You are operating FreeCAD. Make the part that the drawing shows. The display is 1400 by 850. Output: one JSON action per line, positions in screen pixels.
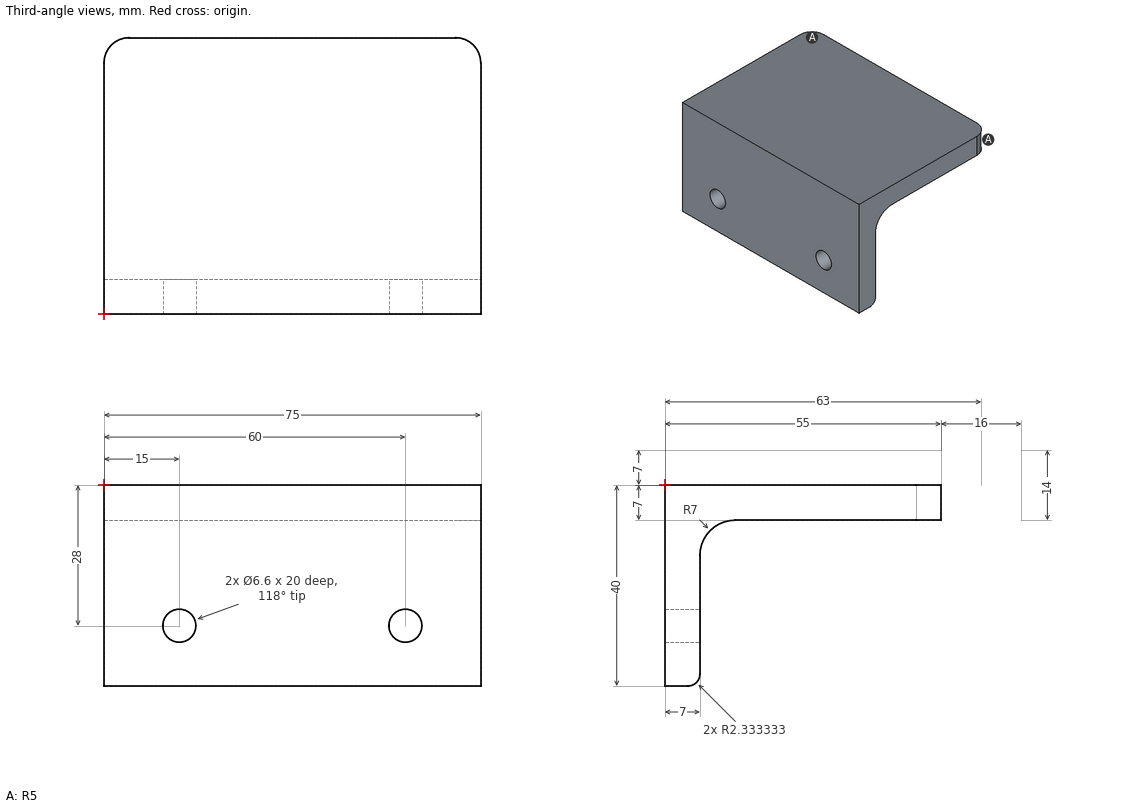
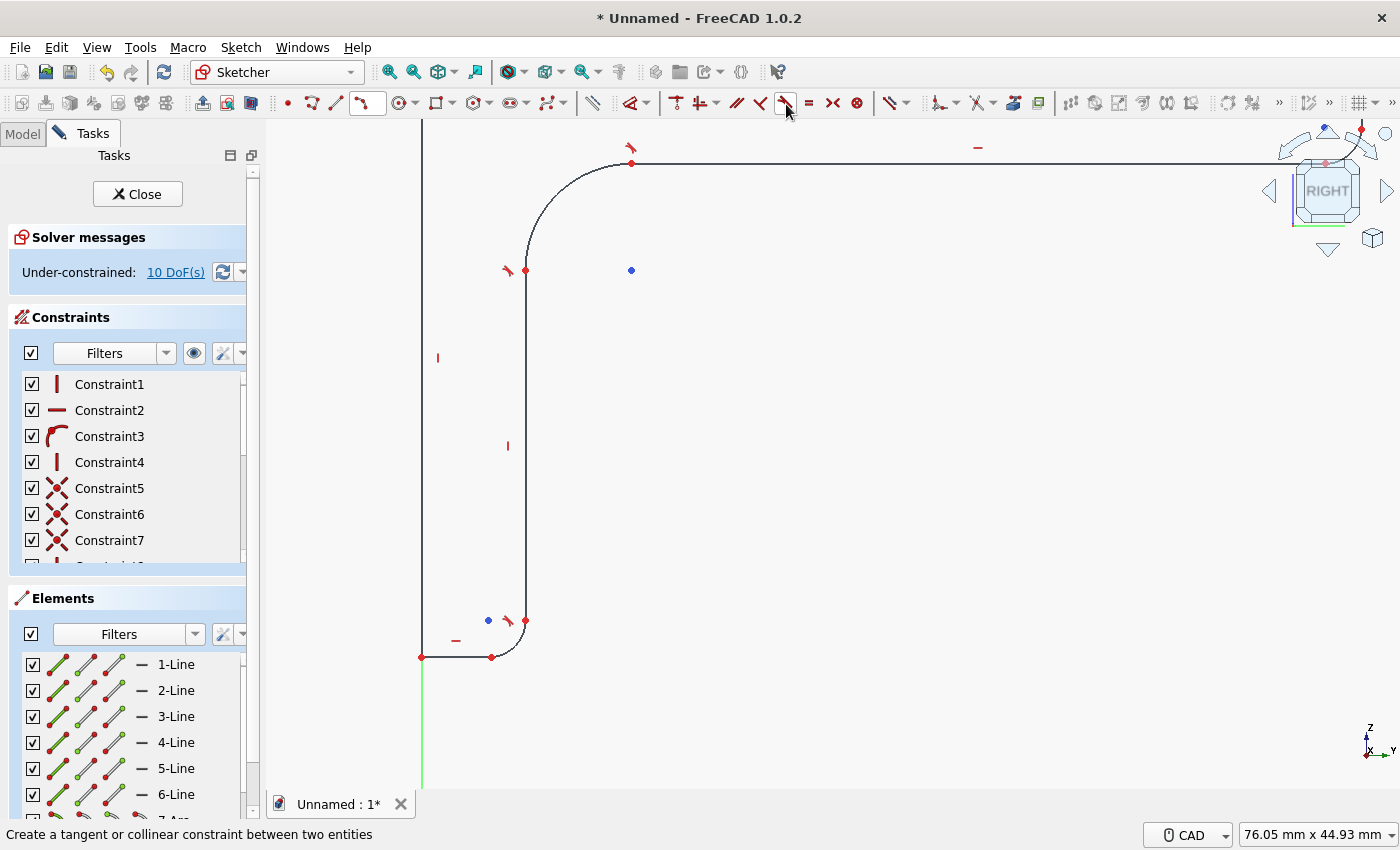
{"action": "left_click", "coordinate": [840, 164]}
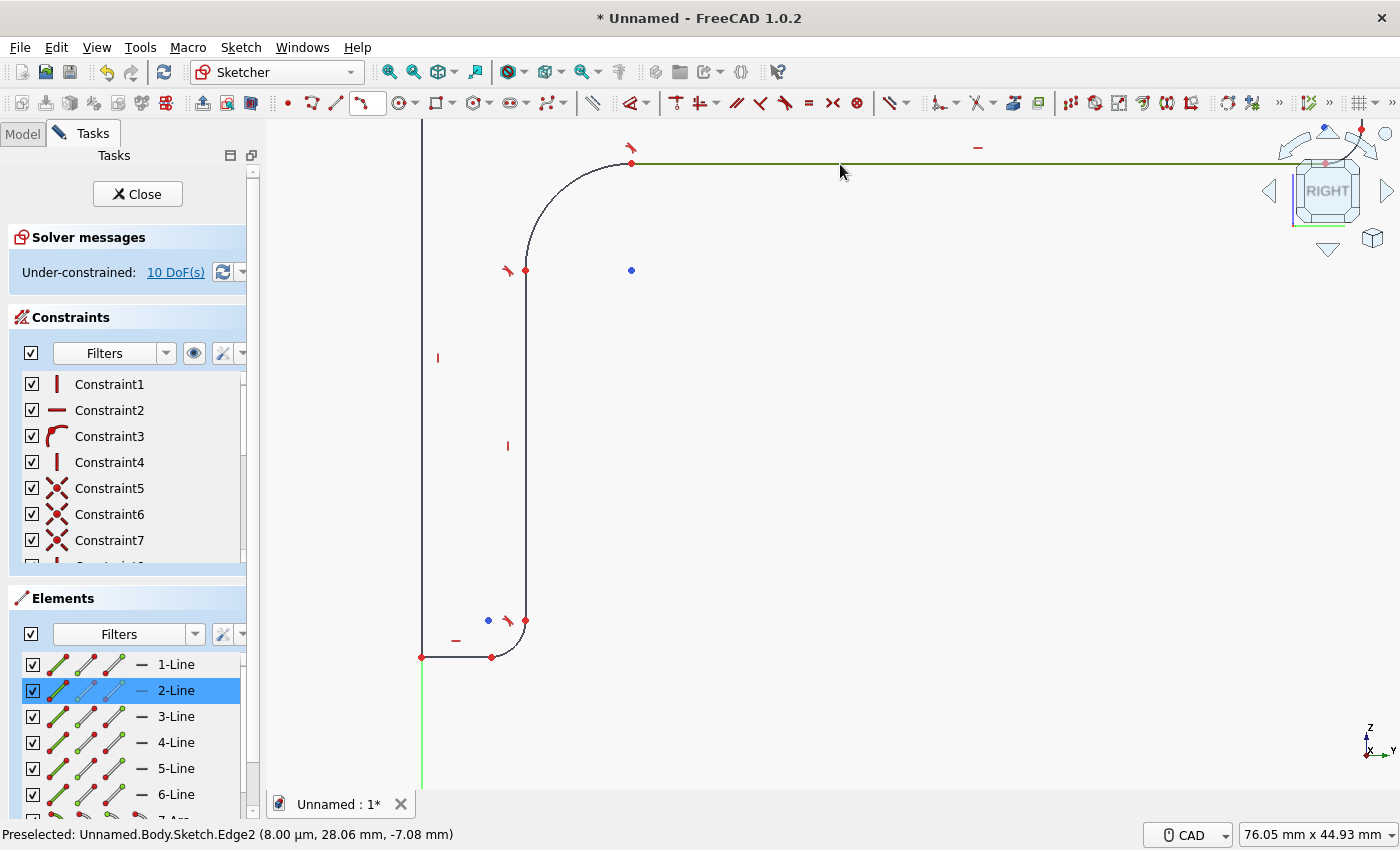
{"action": "scroll", "coordinate": [507, 652], "scroll_direction": "down", "scroll_amount": 2}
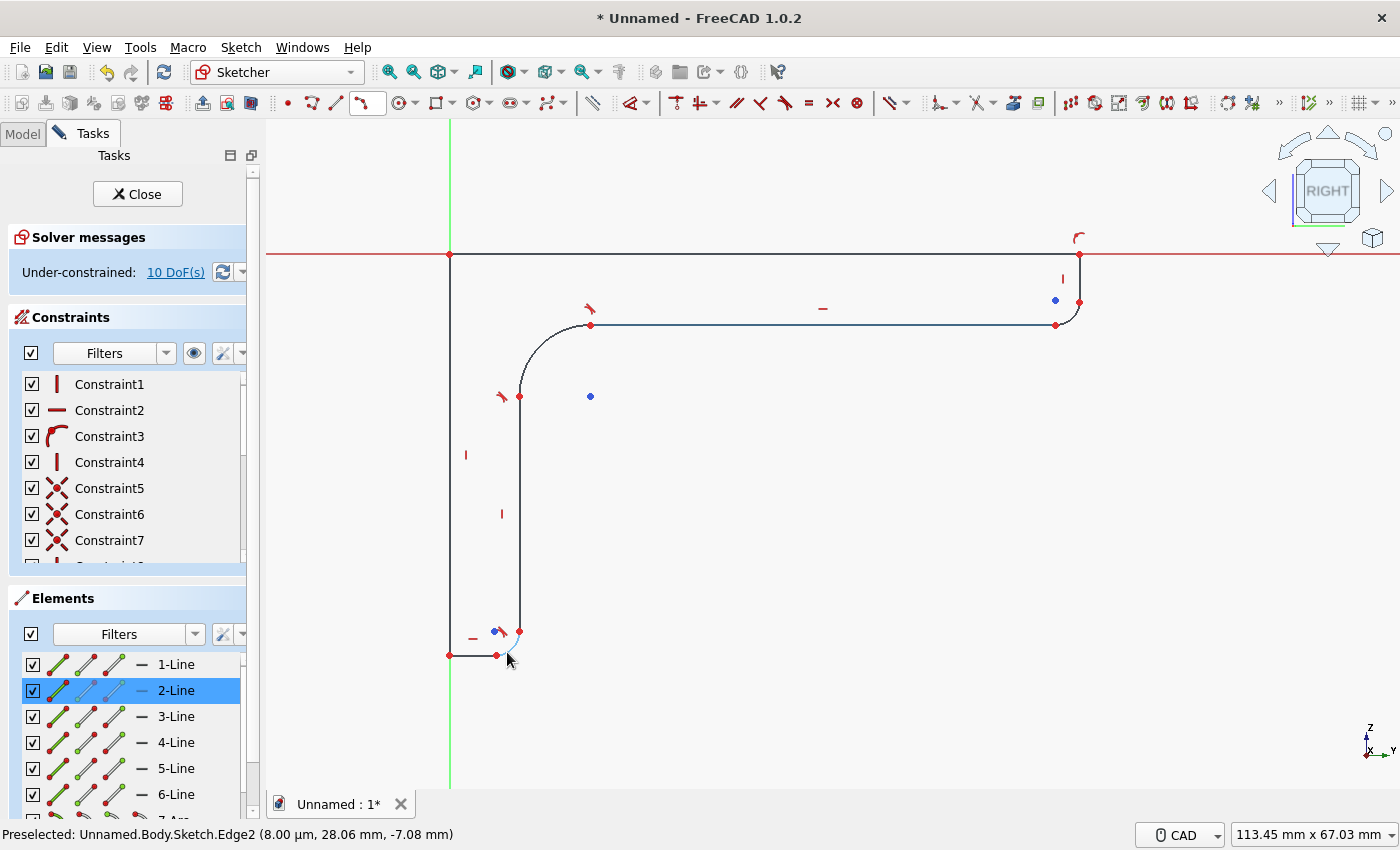
{"action": "scroll", "coordinate": [1066, 322], "scroll_direction": "up", "scroll_amount": 2}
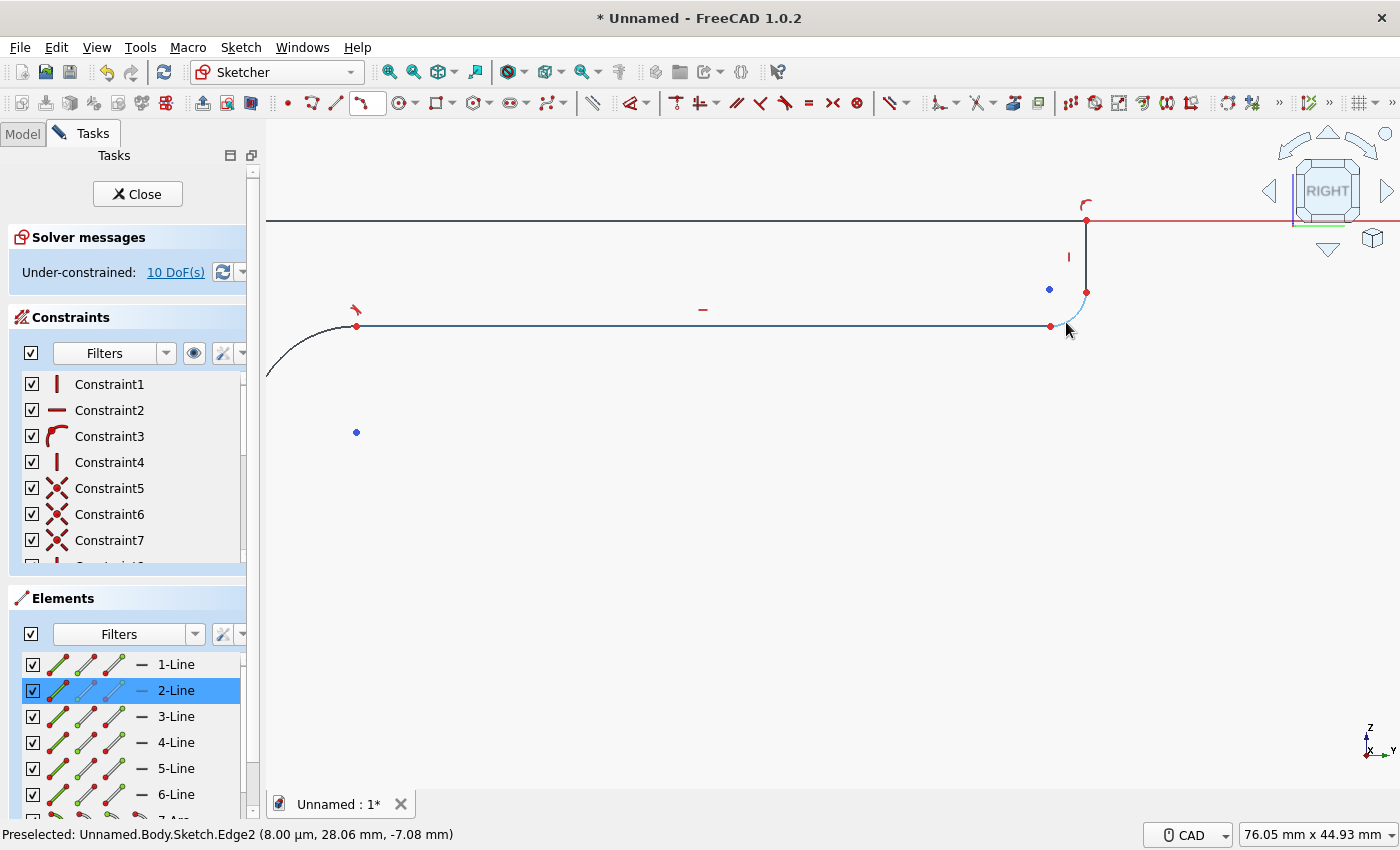
{"action": "left_click", "coordinate": [1066, 322]}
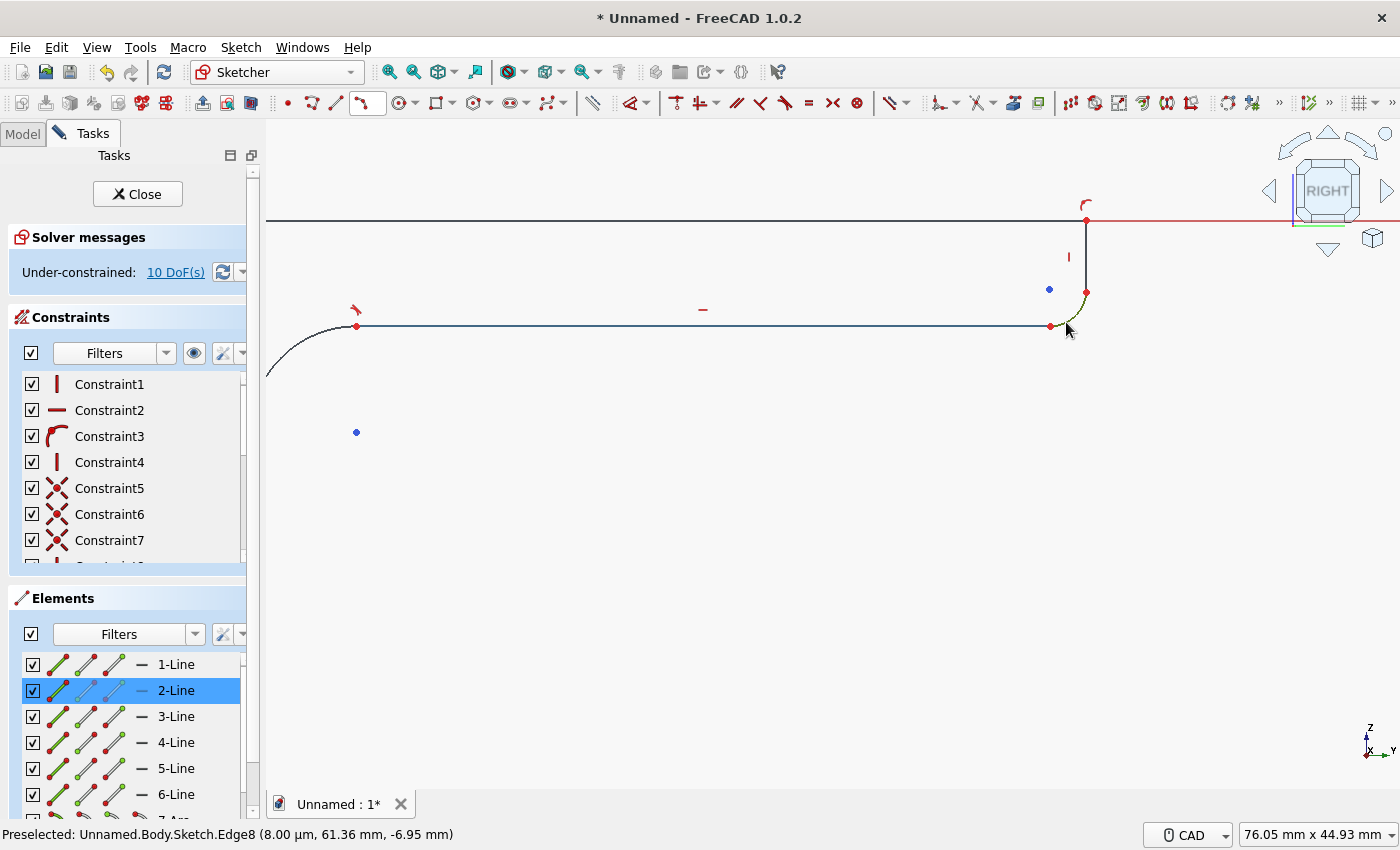
{"action": "left_click", "coordinate": [786, 104]}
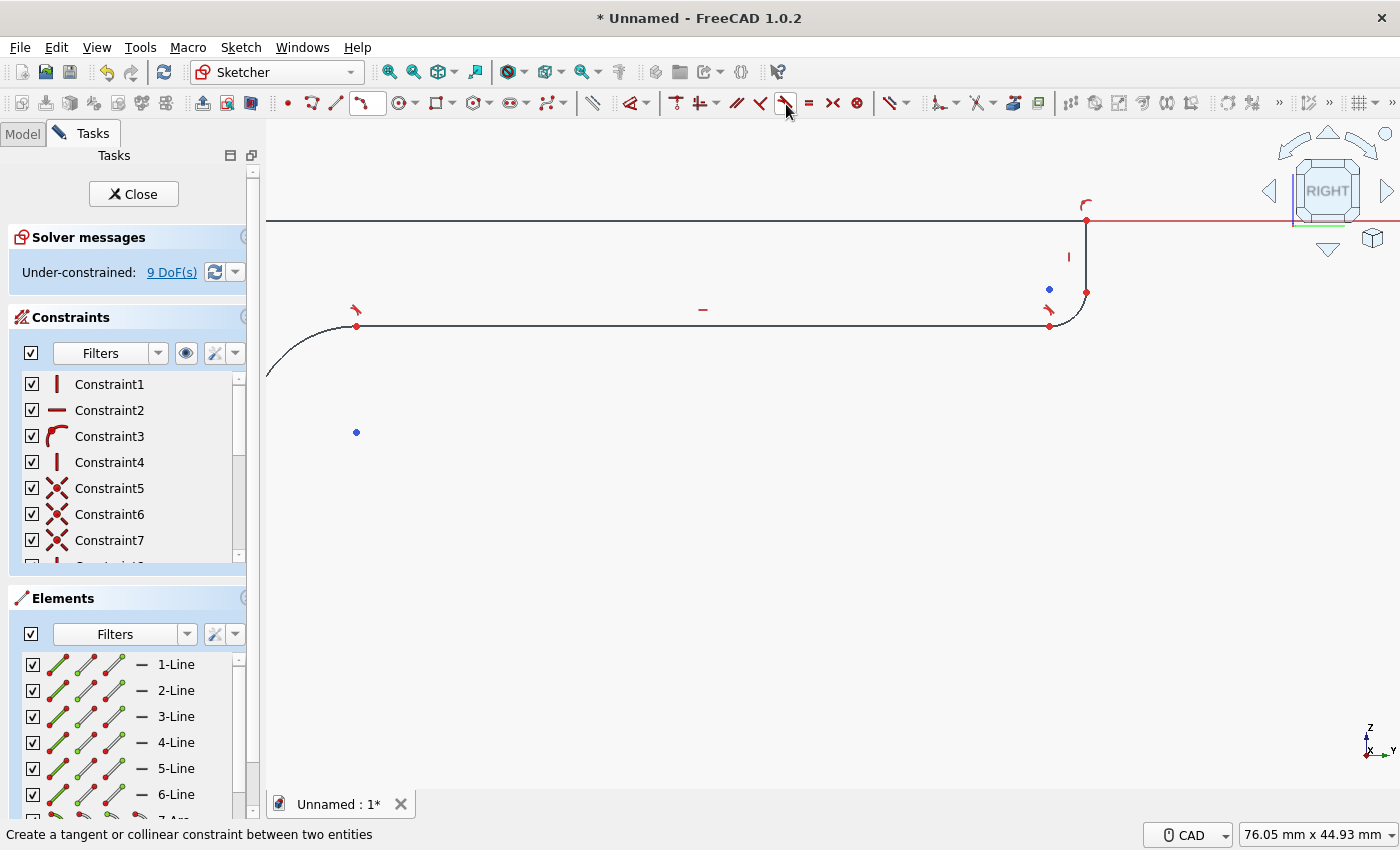
{"action": "left_click", "coordinate": [1086, 271]}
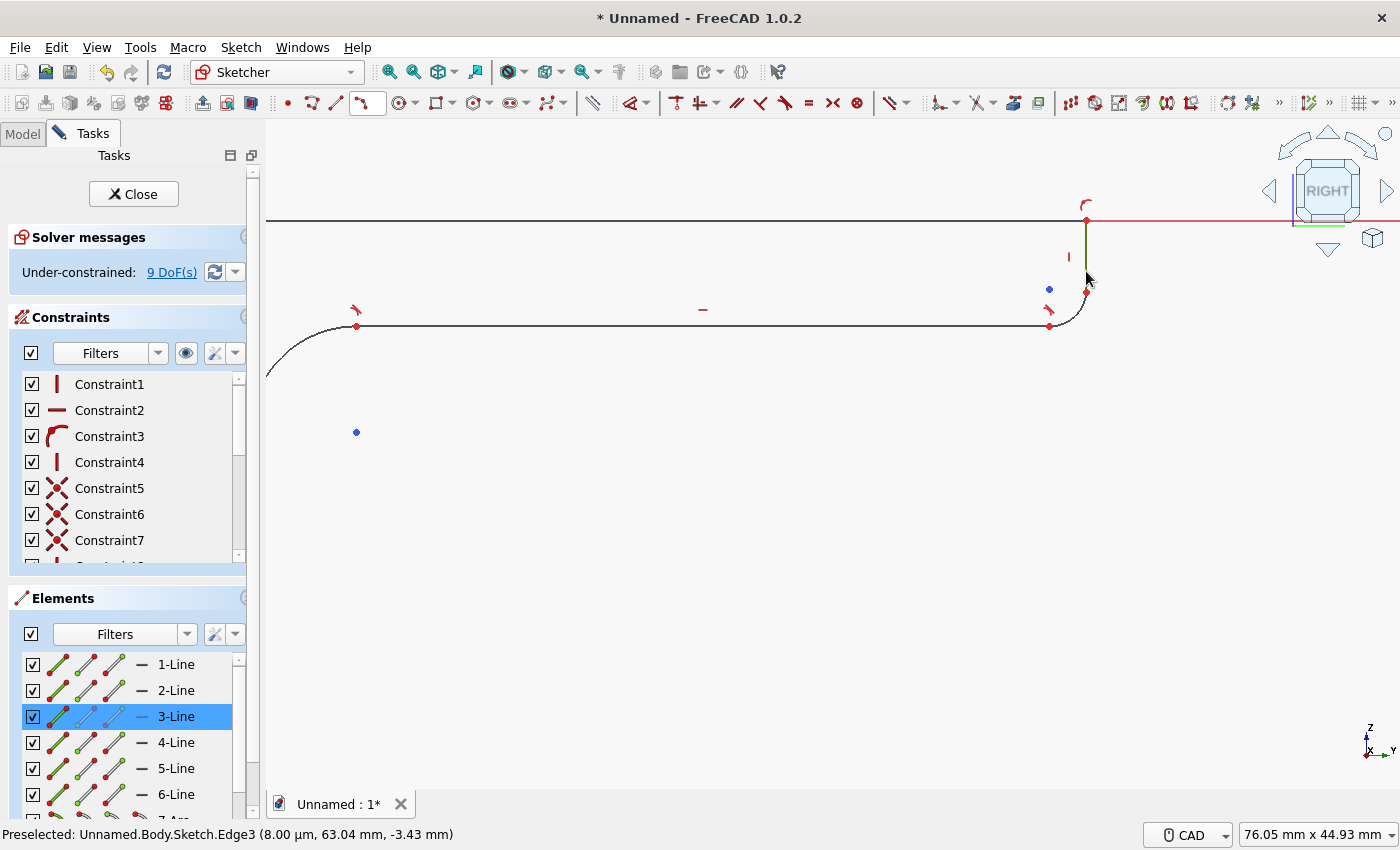
{"action": "left_click", "coordinate": [1066, 323]}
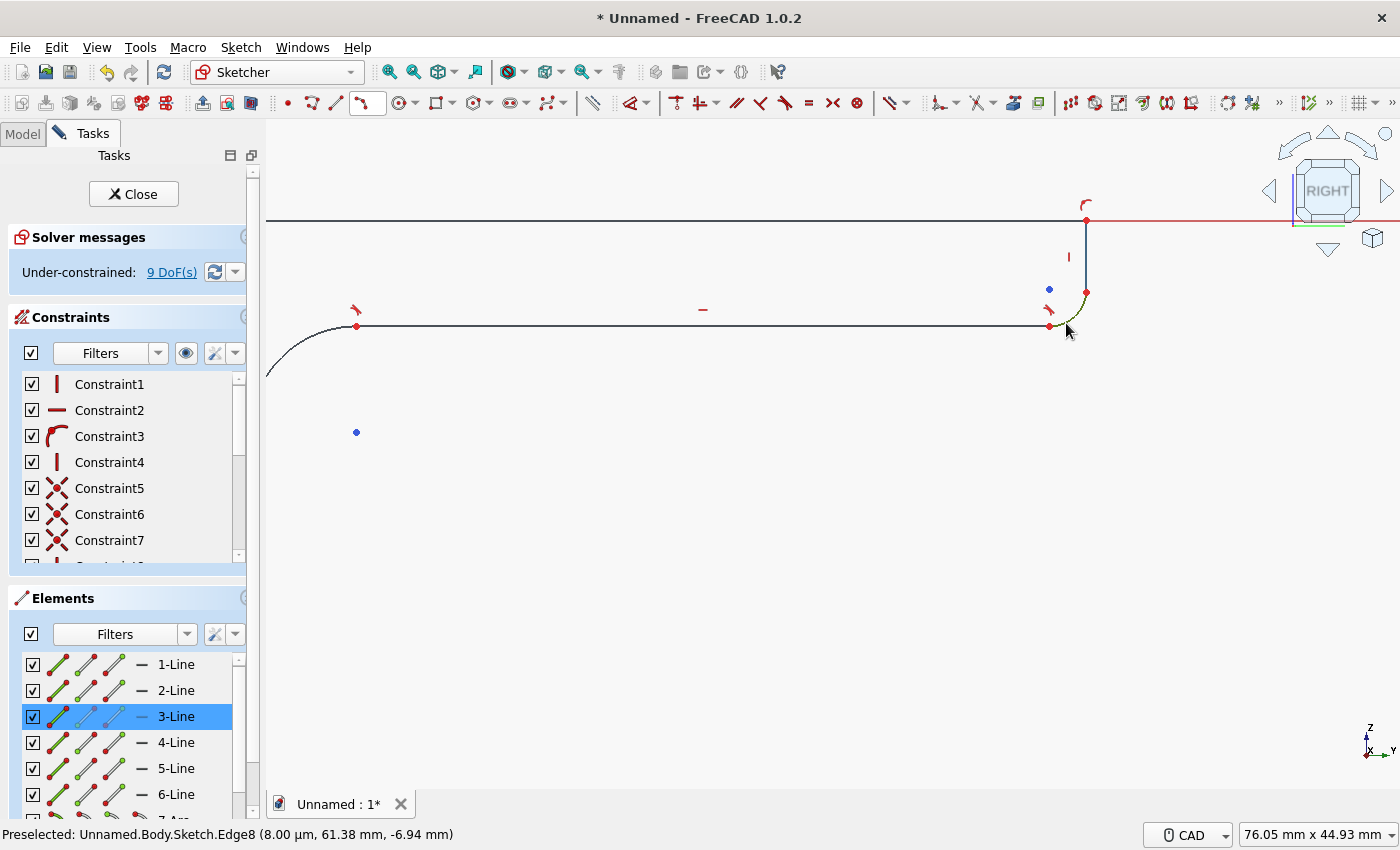
{"action": "left_click", "coordinate": [786, 104]}